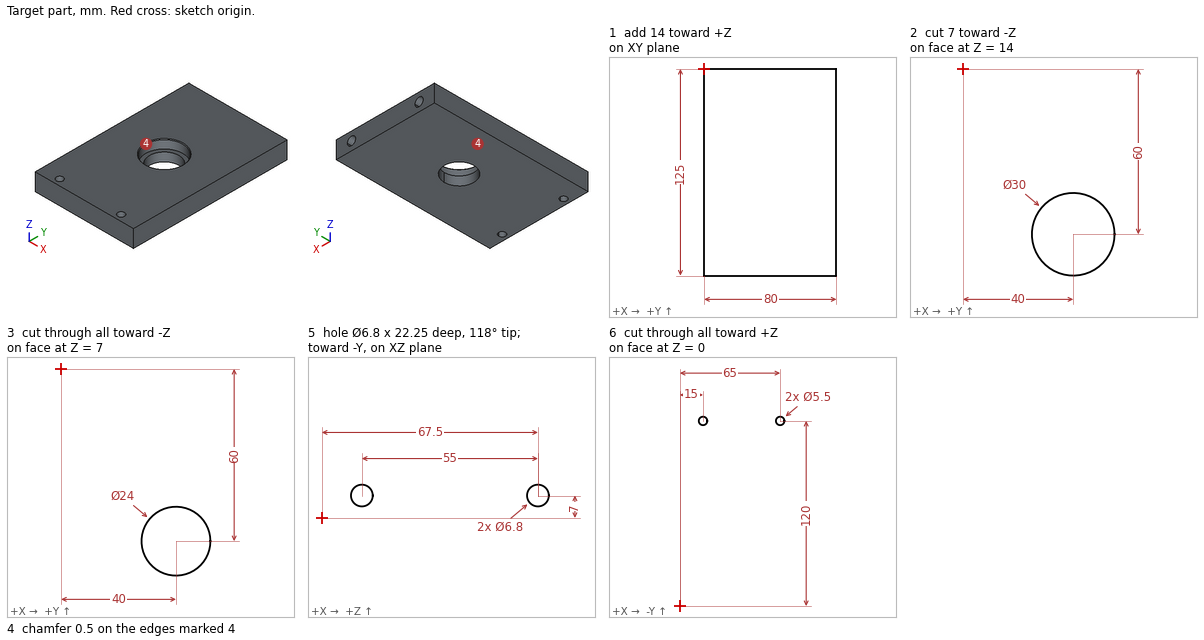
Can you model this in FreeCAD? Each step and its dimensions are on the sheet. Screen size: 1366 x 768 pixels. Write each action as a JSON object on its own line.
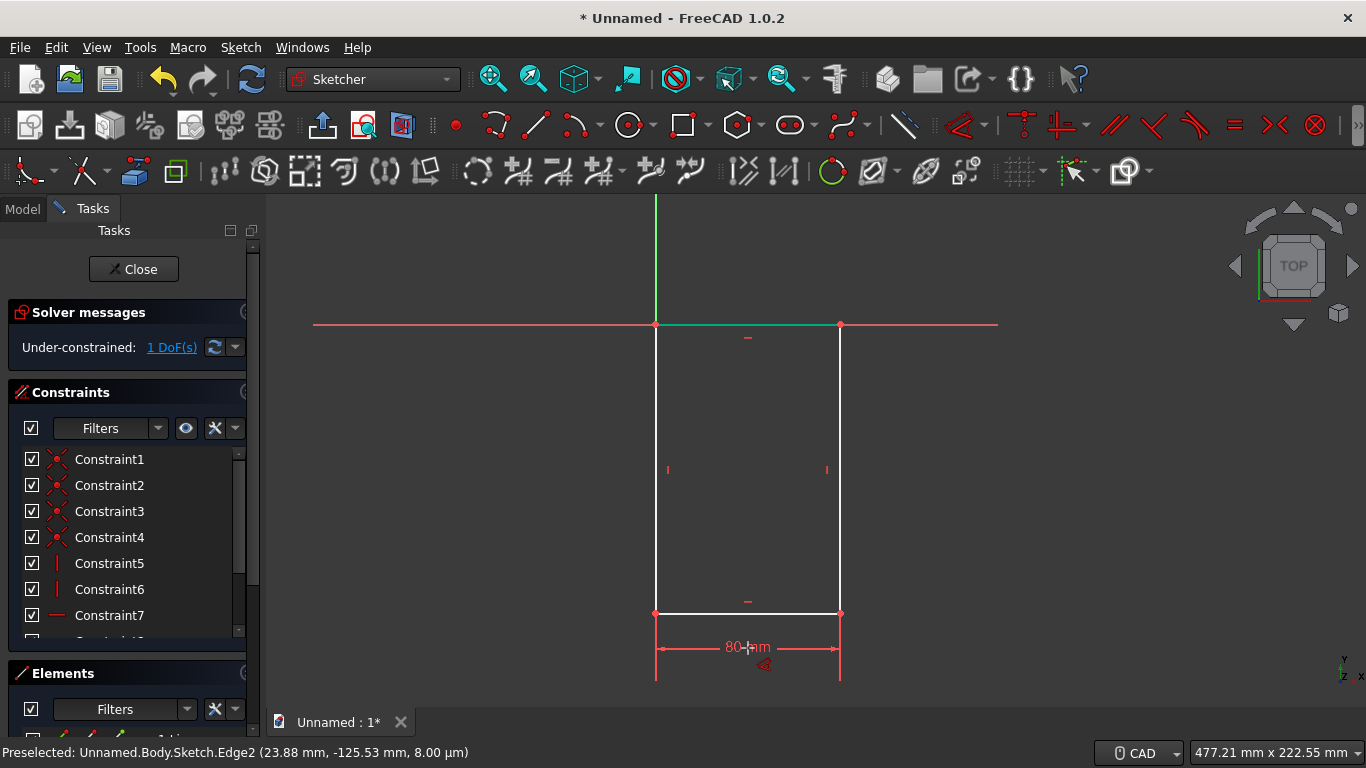
{"action": "left_click", "coordinate": [656, 411]}
{"action": "left_click", "coordinate": [622, 469]}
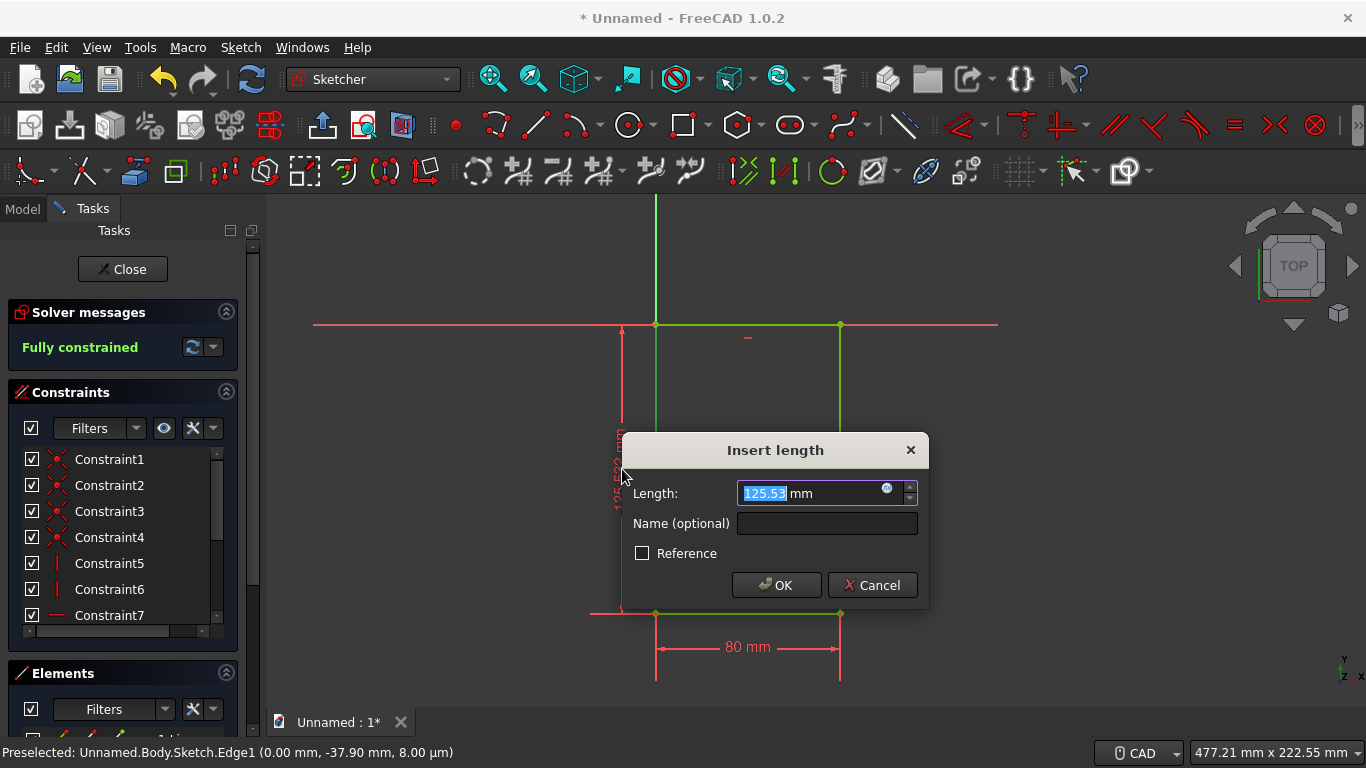
{"action": "type", "text": "125"}
{"action": "key", "text": "Return"}
{"action": "key", "text": "Escape"}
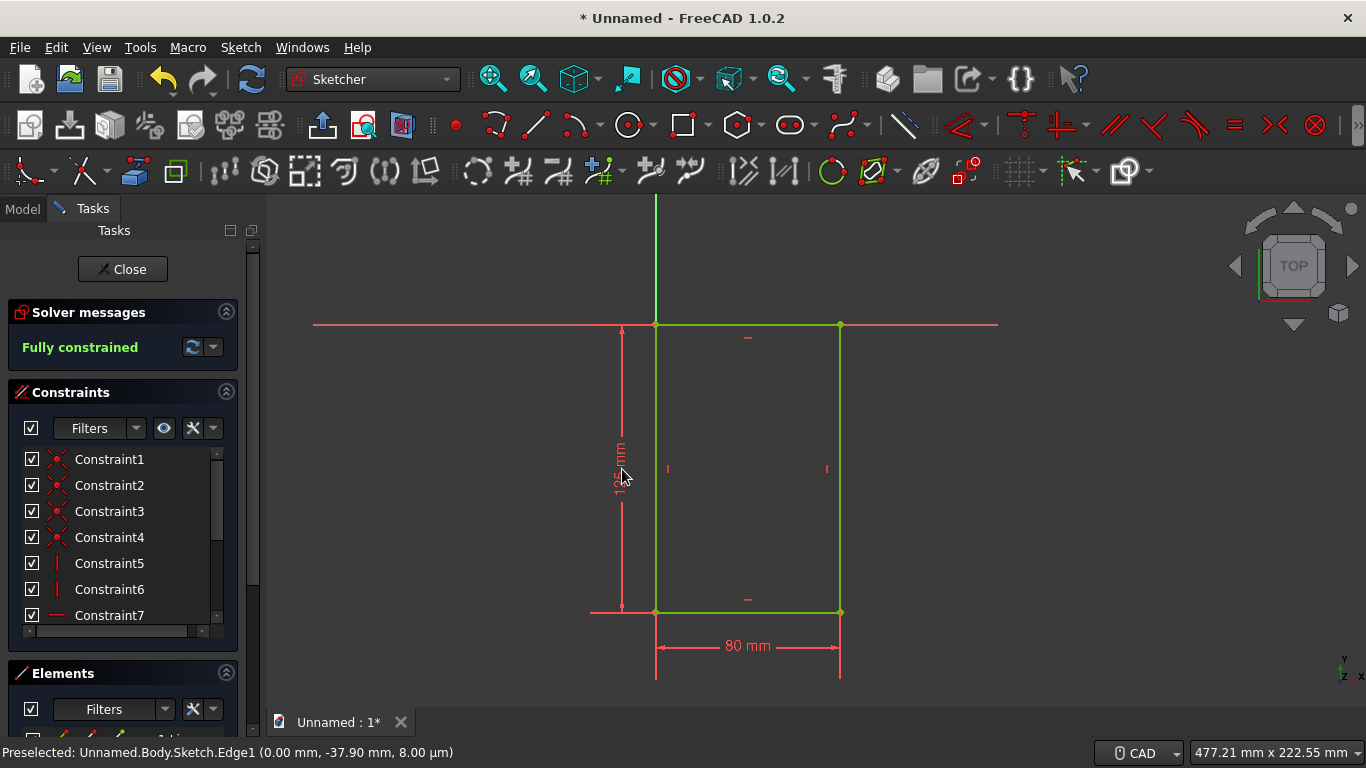
{"action": "left_click", "coordinate": [123, 269]}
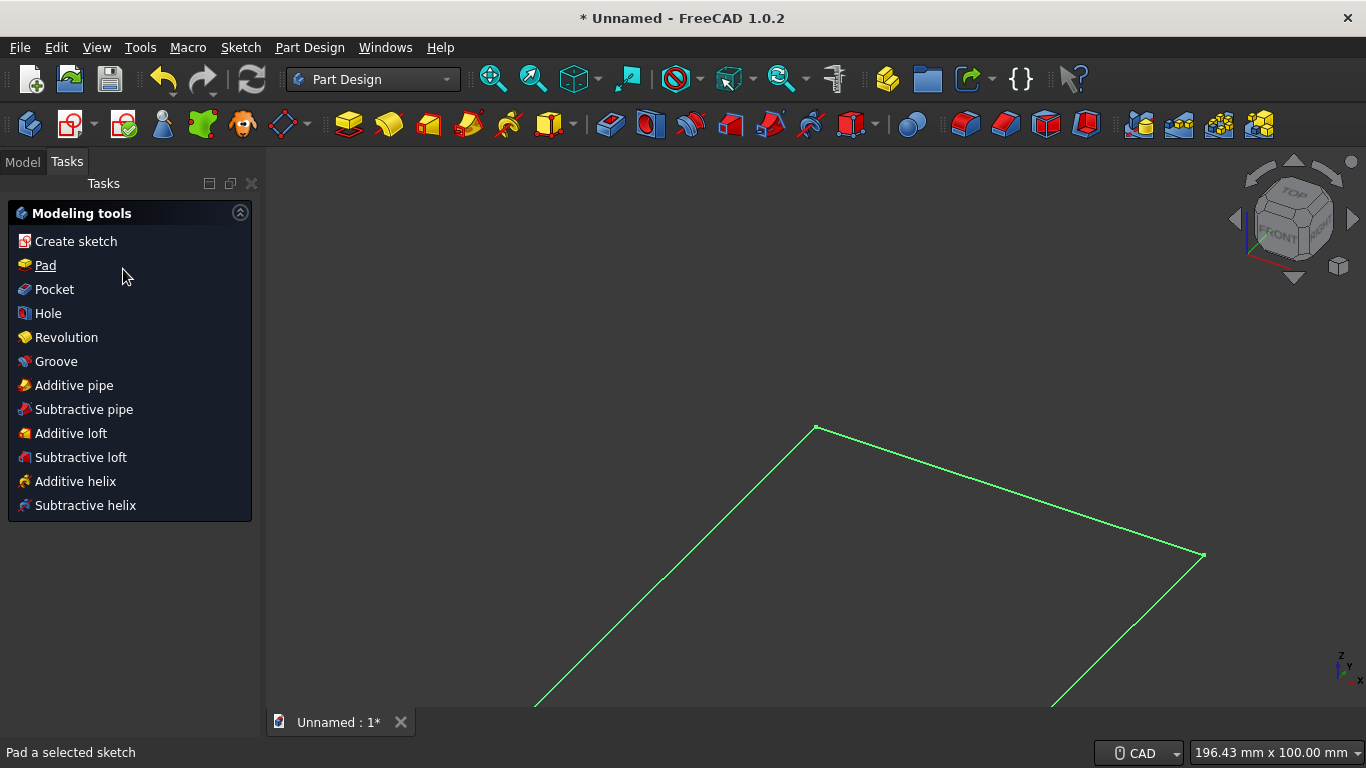
{"action": "left_click", "coordinate": [350, 124]}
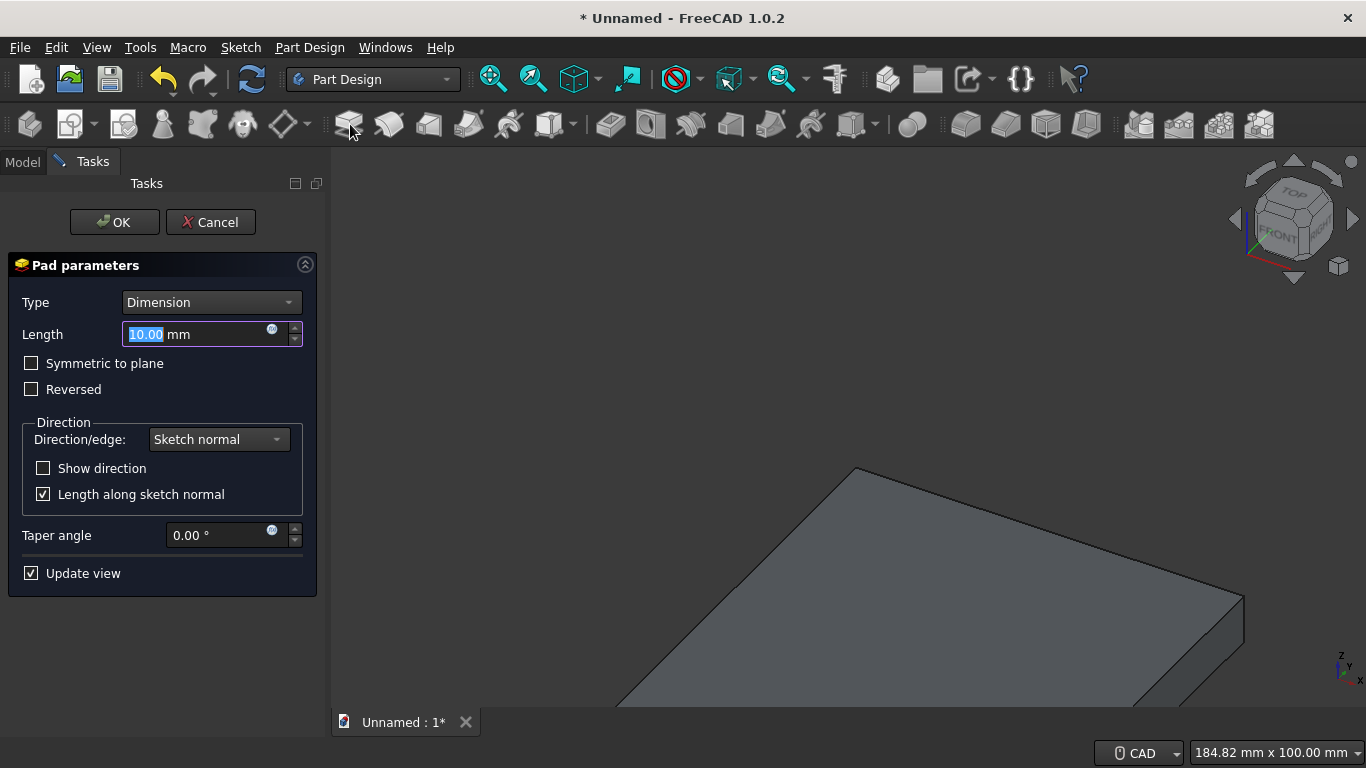
{"action": "type", "text": "14"}
{"action": "key", "text": "Tab"}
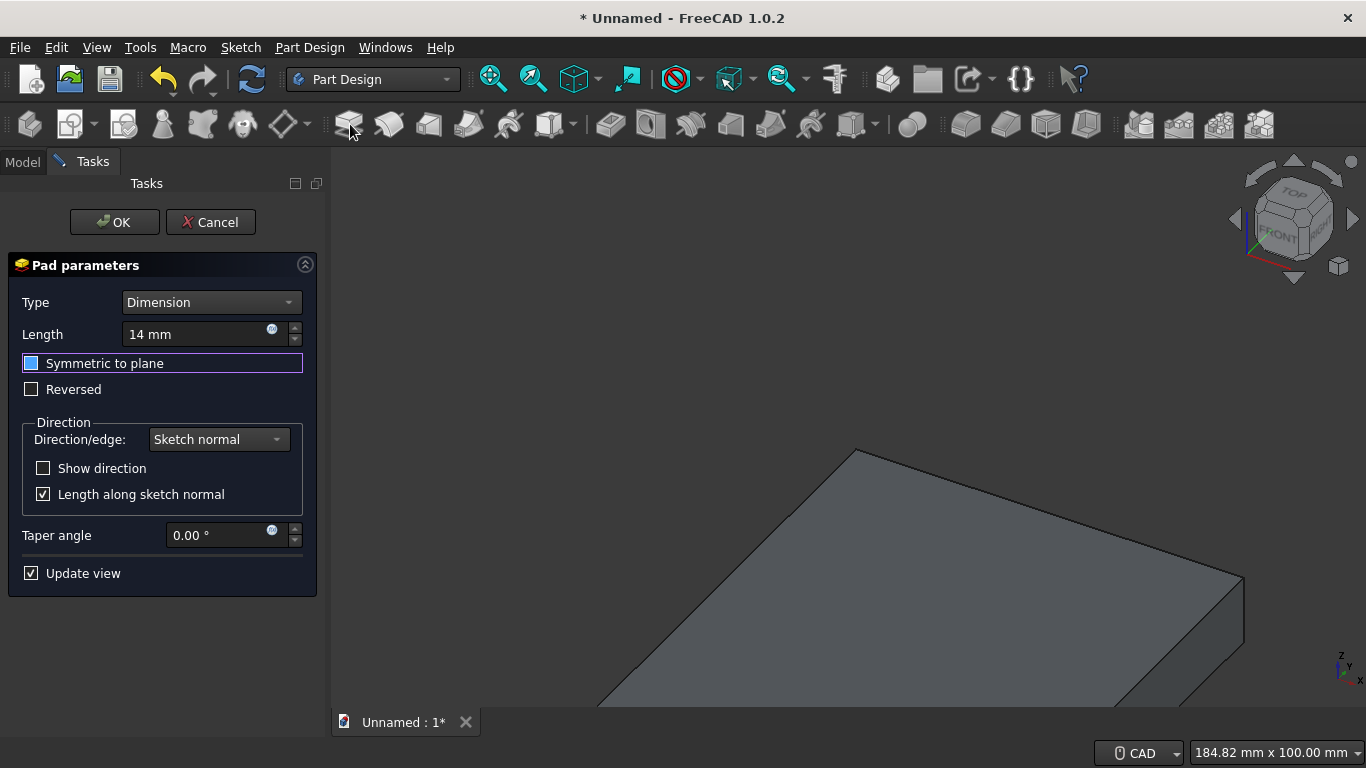
{"action": "left_click", "coordinate": [115, 222]}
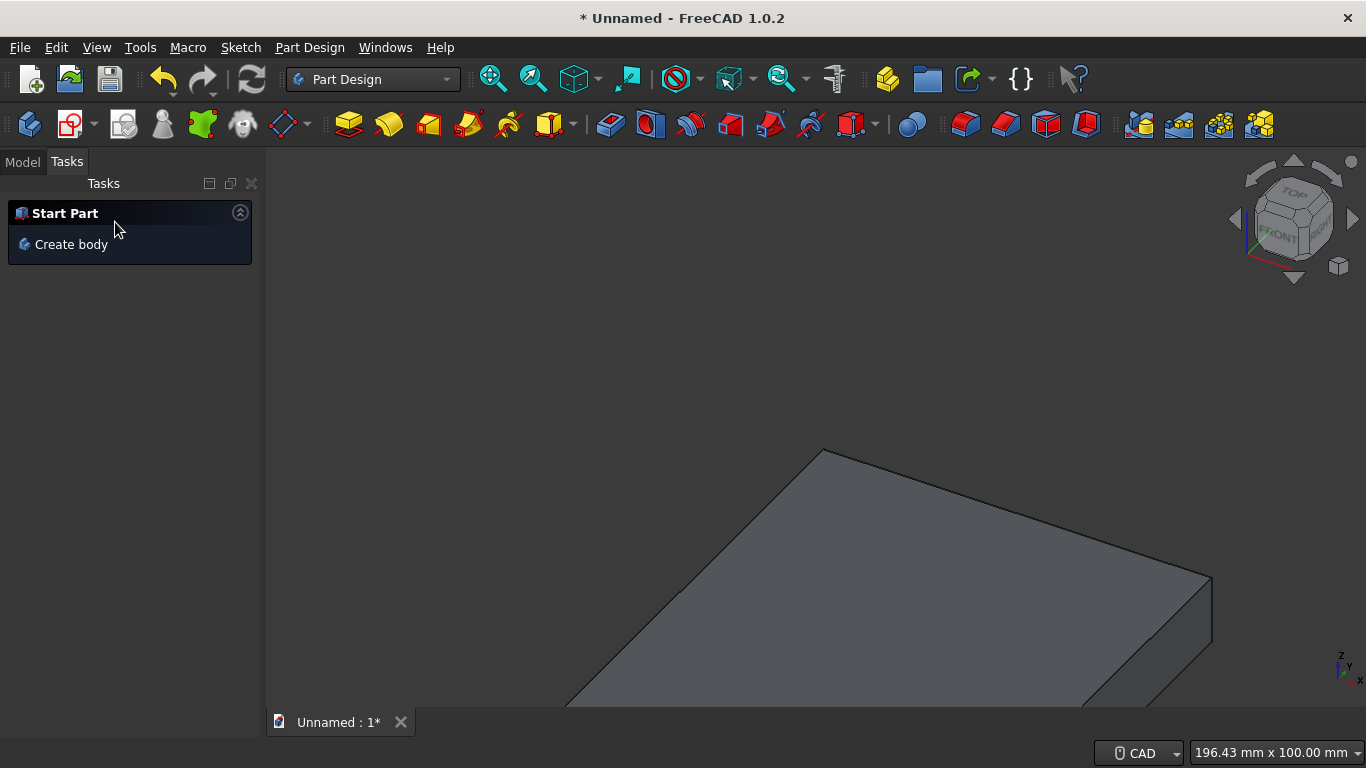
{"action": "left_click", "coordinate": [494, 80]}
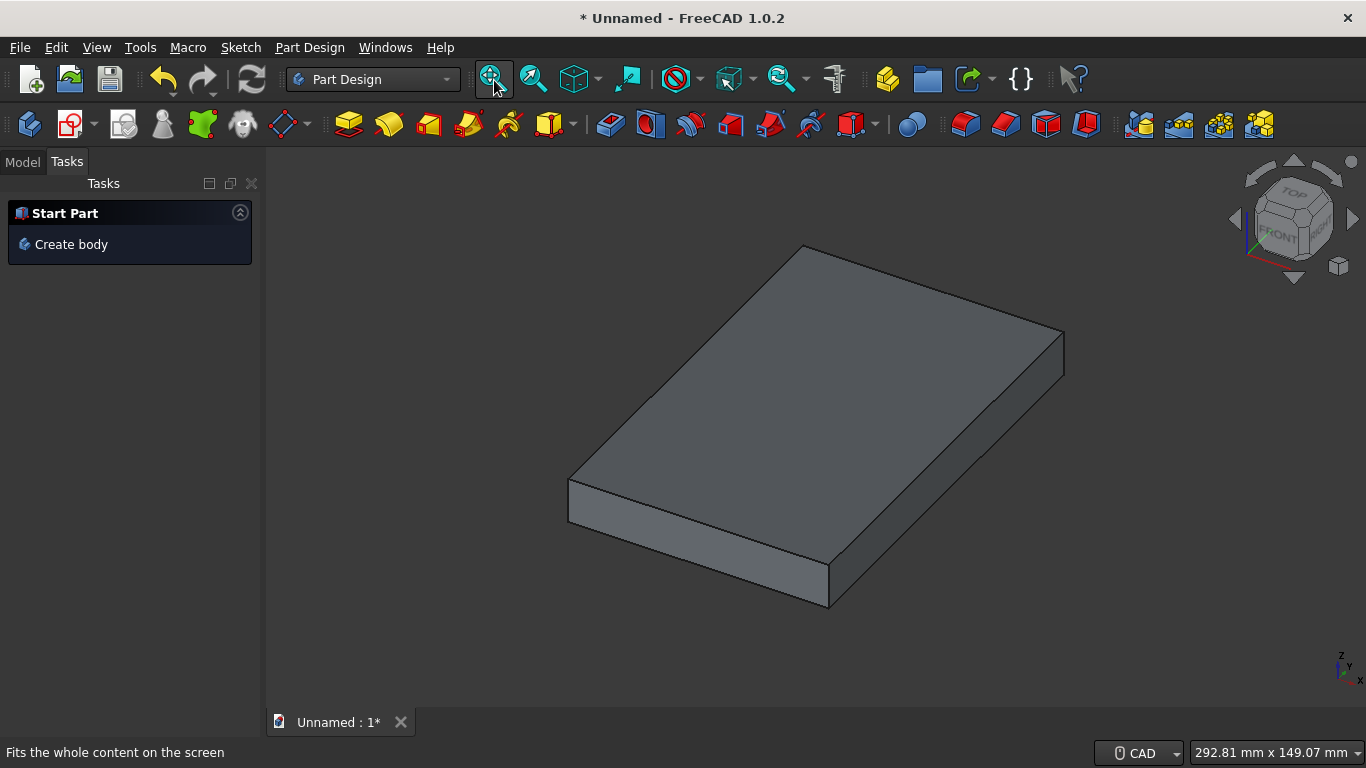
{"action": "left_click", "coordinate": [850, 371]}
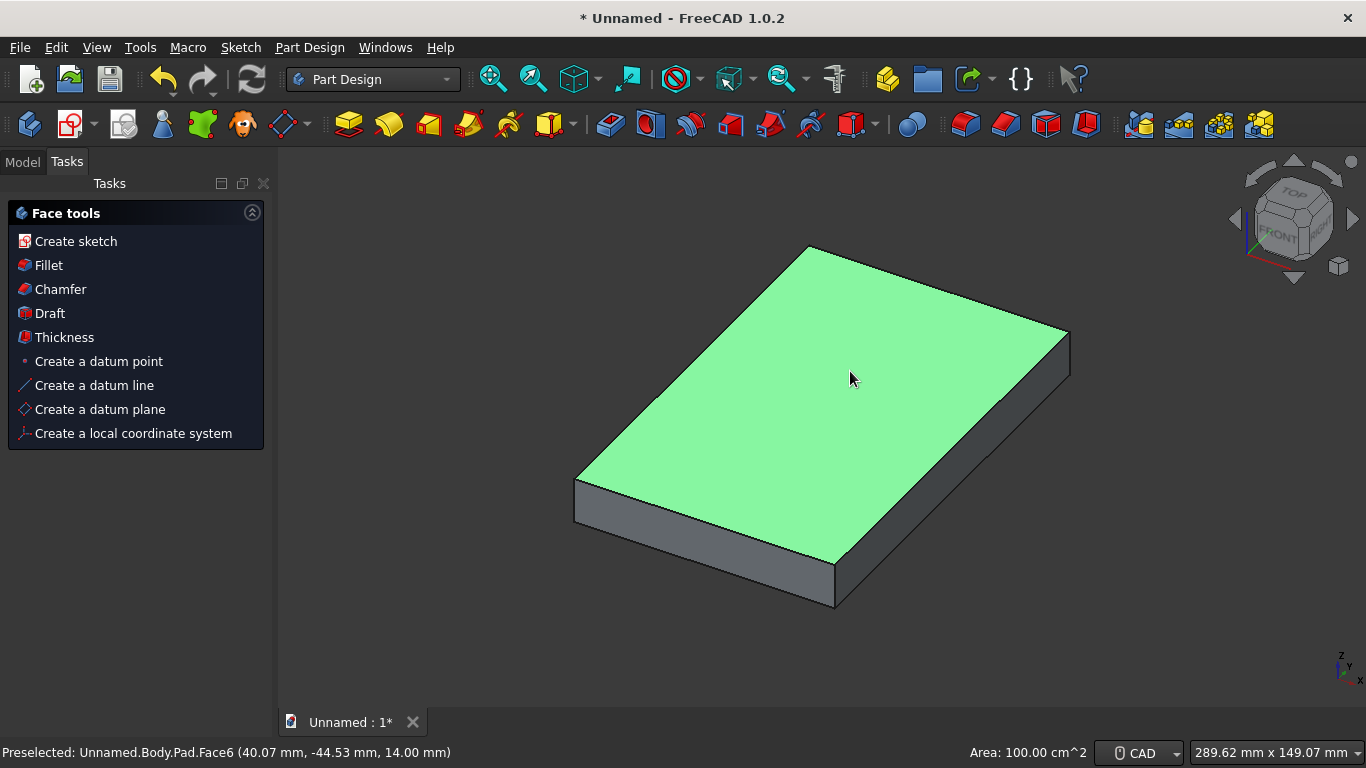
{"action": "left_click", "coordinate": [70, 124]}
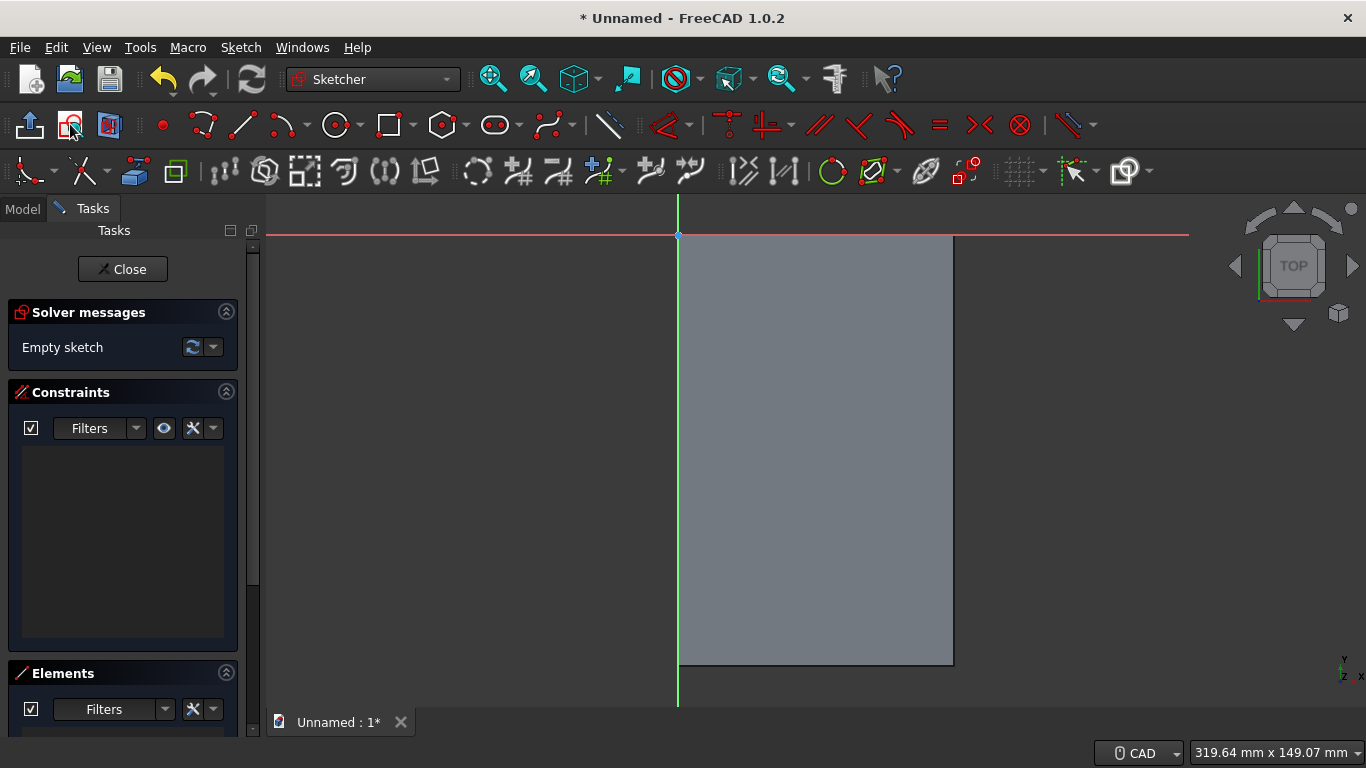
{"action": "scroll", "coordinate": [846, 438], "scroll_direction": "up", "scroll_amount": 6}